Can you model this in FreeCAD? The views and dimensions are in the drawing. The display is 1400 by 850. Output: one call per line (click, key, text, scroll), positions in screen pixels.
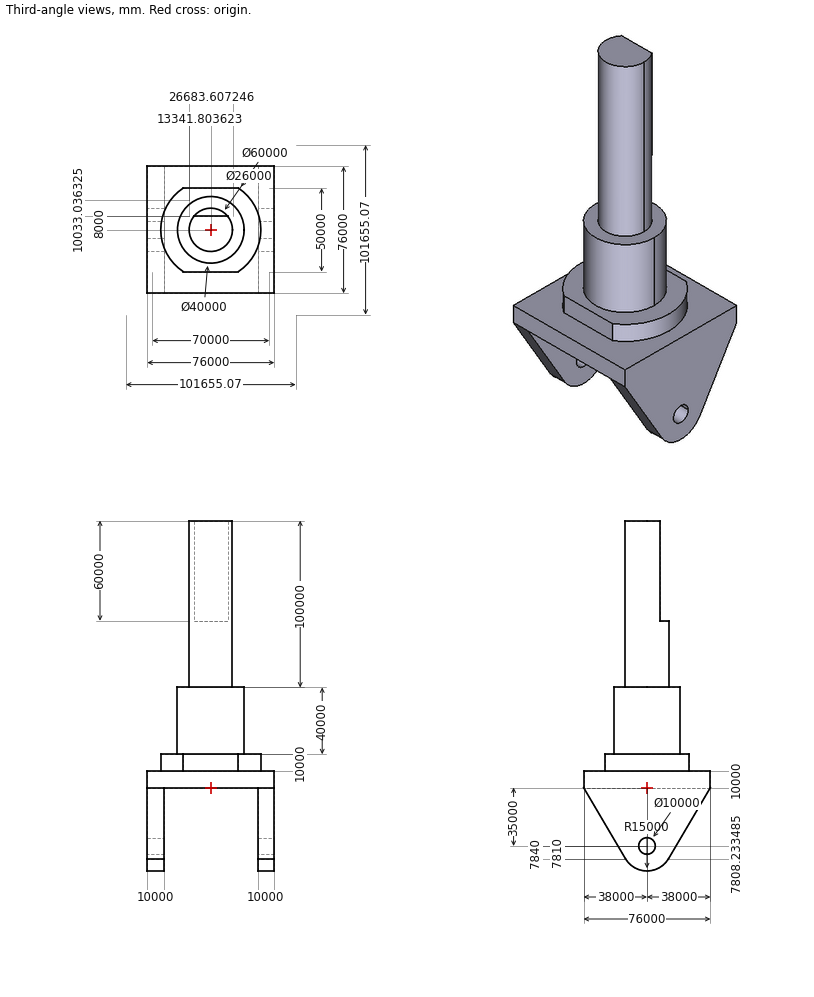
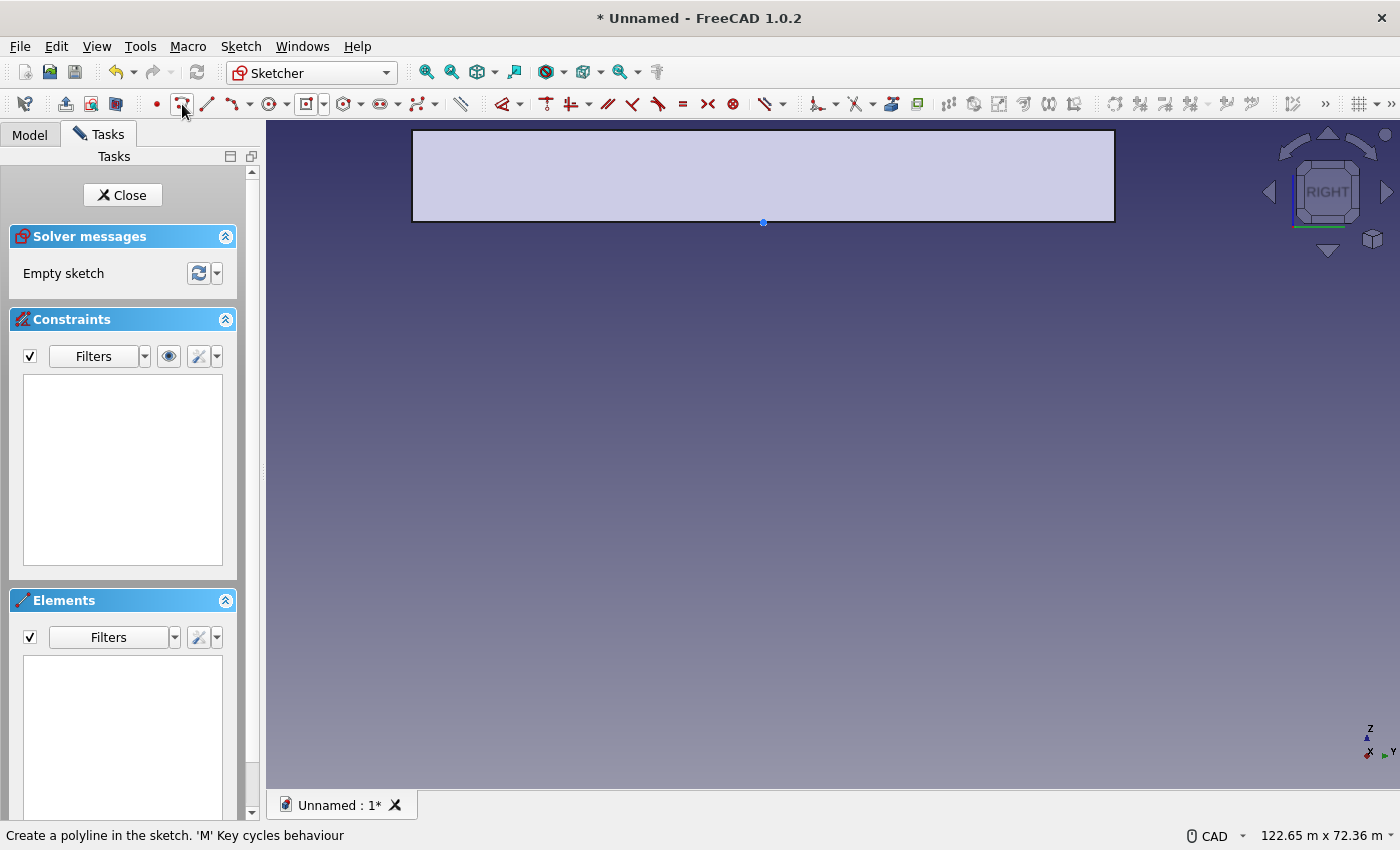
click(882, 618)
click(1115, 222)
click(412, 231)
click(645, 618)
right_click(645, 618)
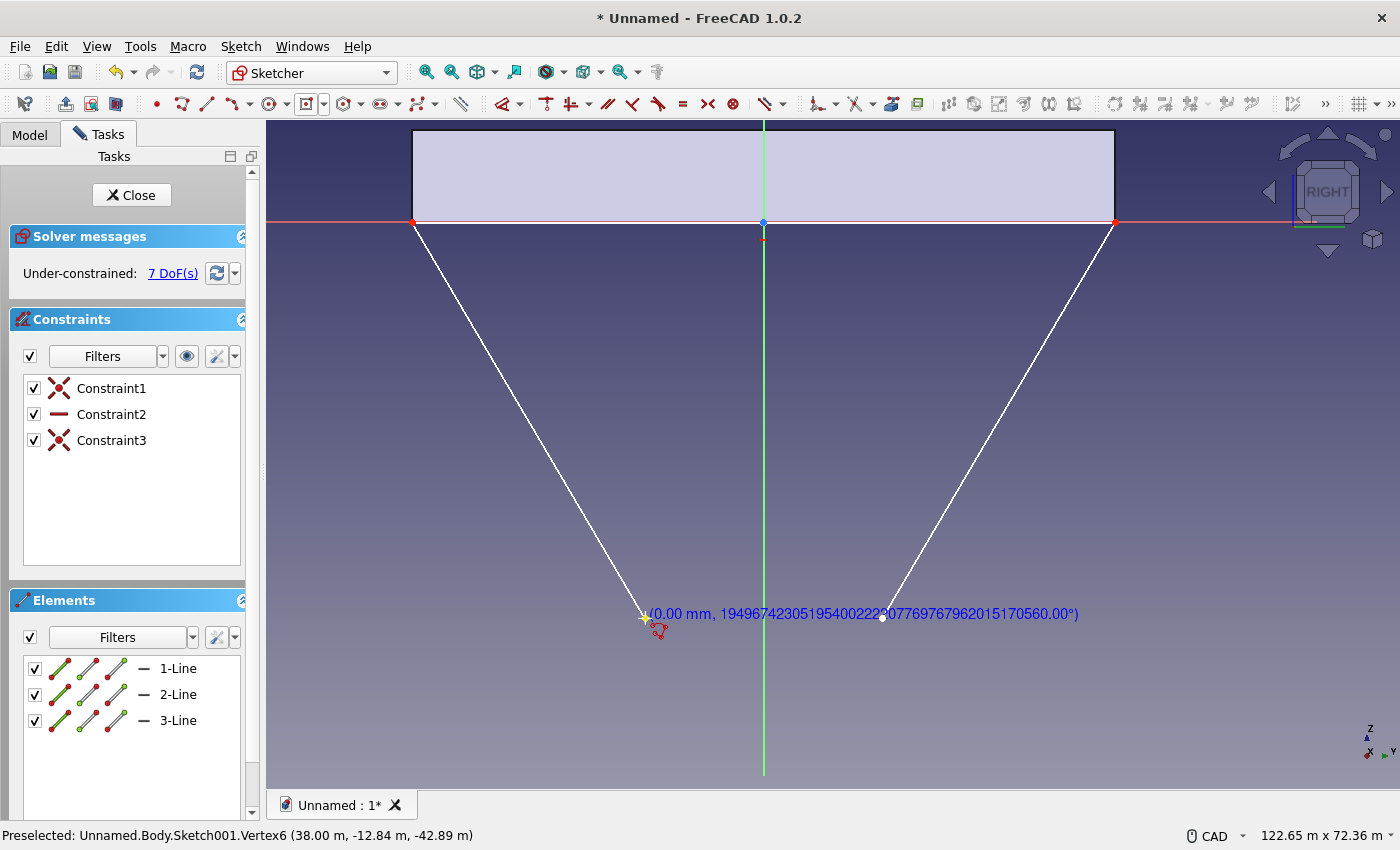
click(232, 104)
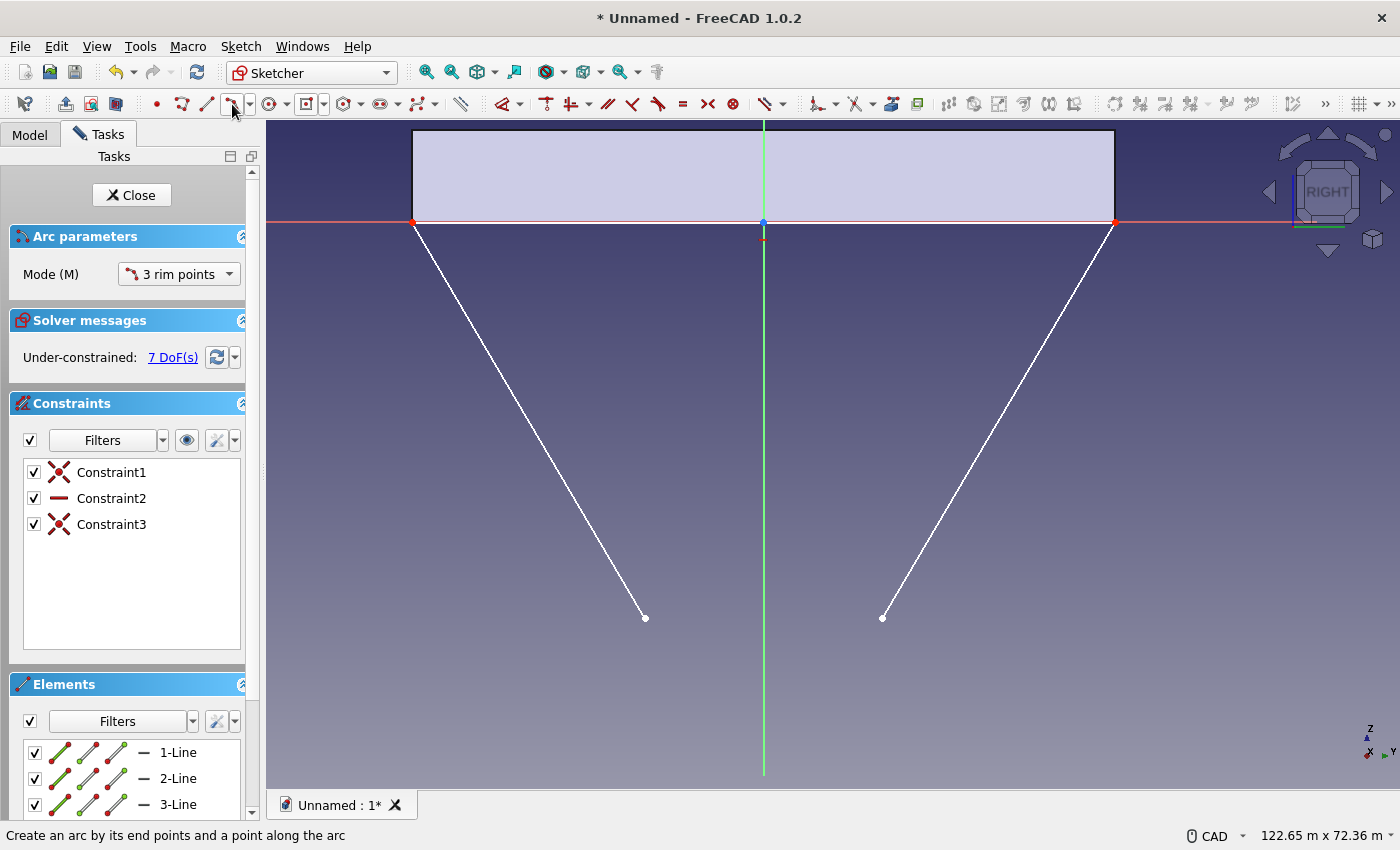
click(645, 619)
click(882, 619)
click(736, 682)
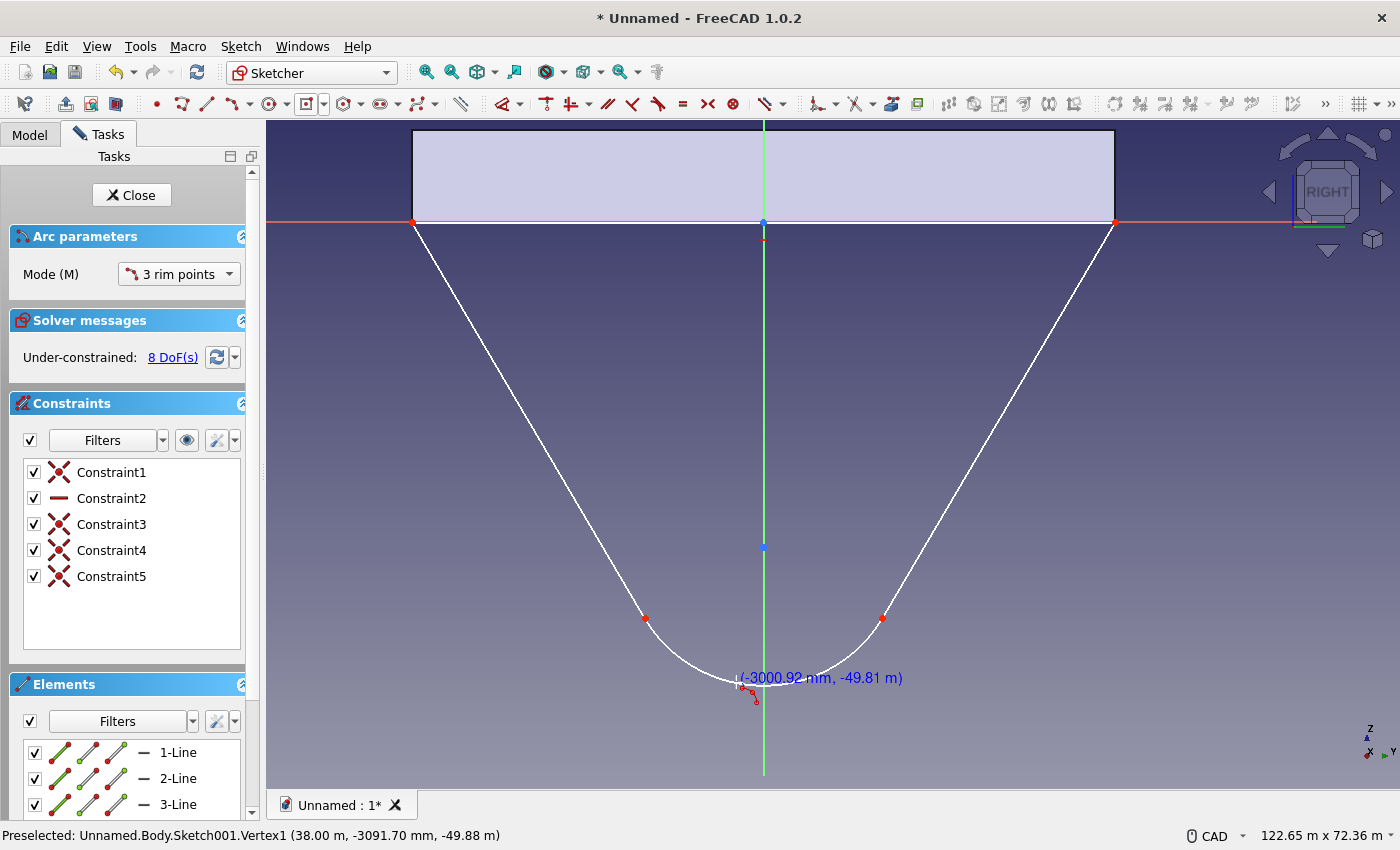
click(268, 104)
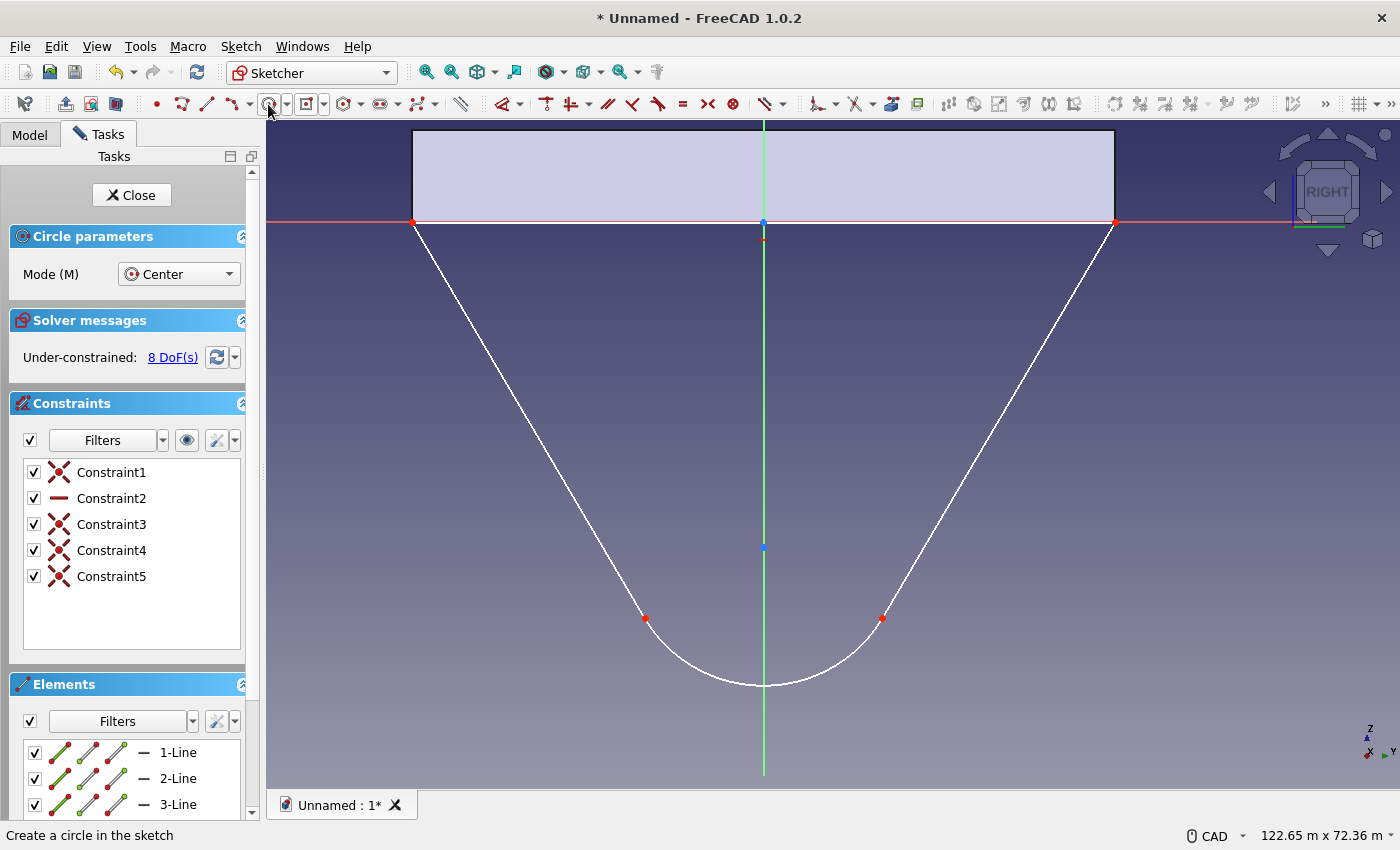
click(764, 546)
click(796, 513)
key(Escape)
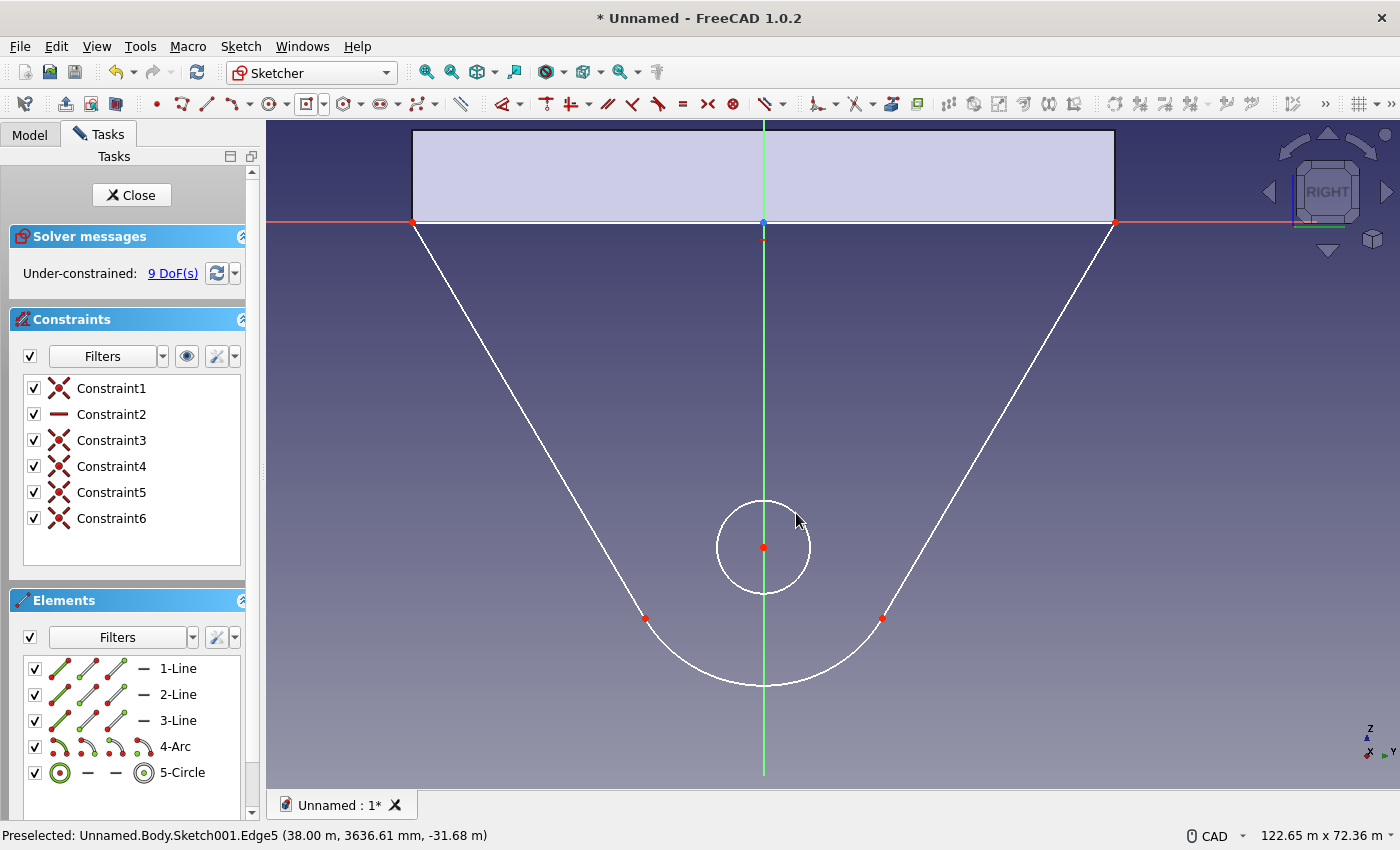
click(763, 547)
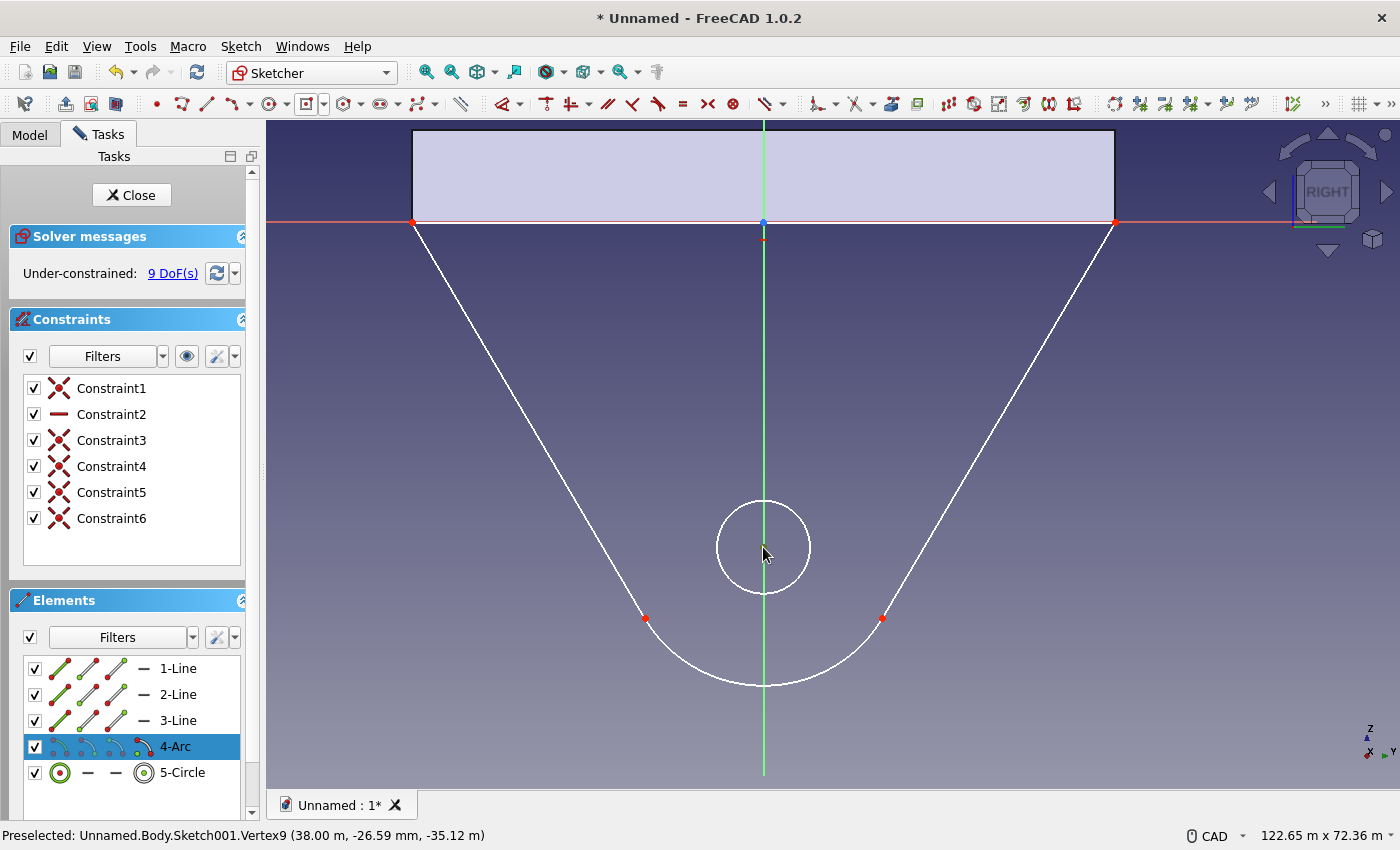
click(764, 717)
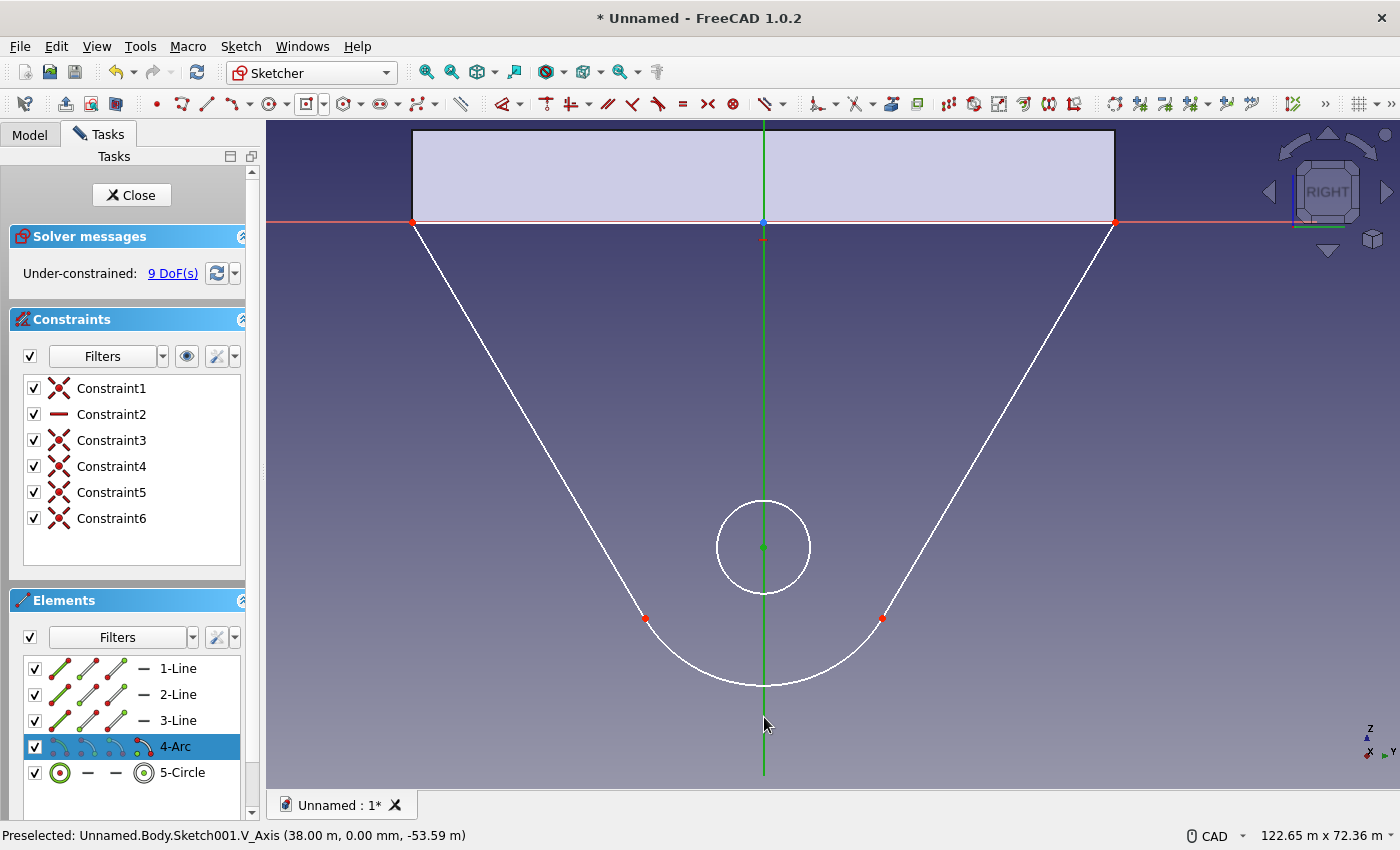
click(546, 104)